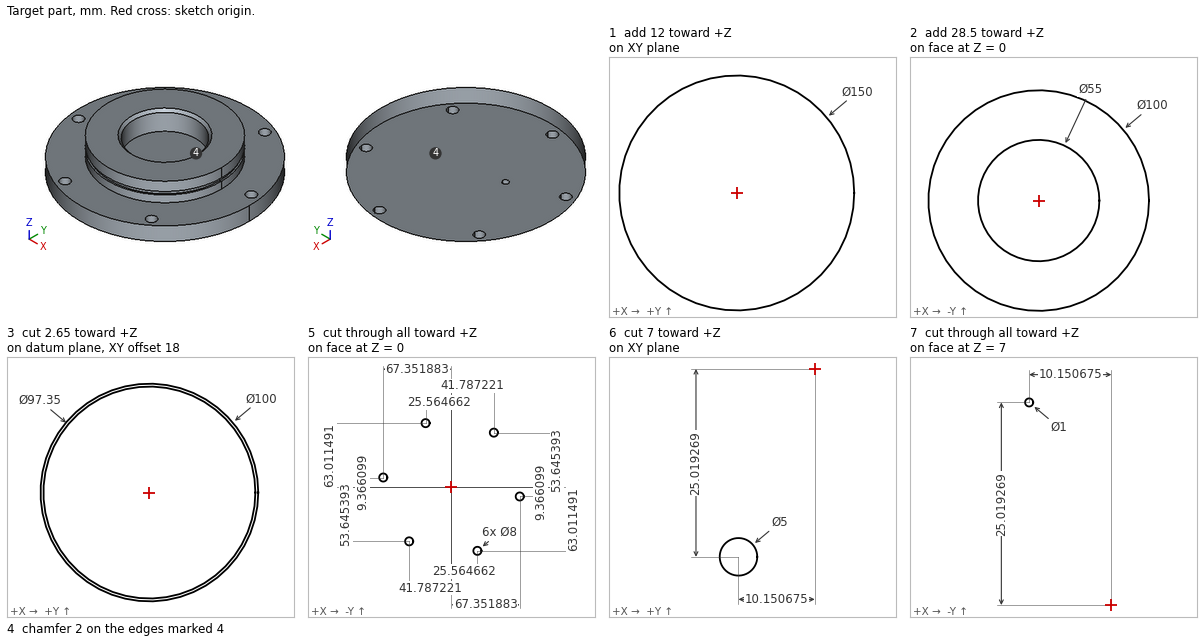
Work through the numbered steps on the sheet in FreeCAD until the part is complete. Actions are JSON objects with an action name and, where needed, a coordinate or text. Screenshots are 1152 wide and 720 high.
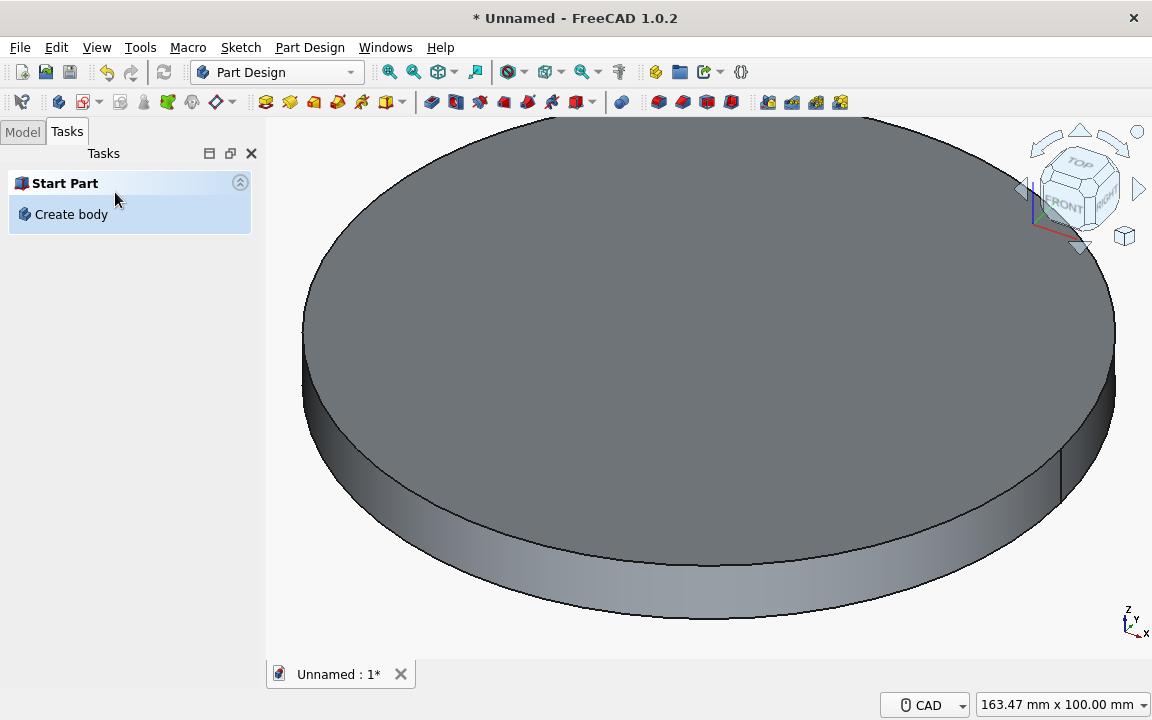
{"action": "left_click", "coordinate": [390, 72]}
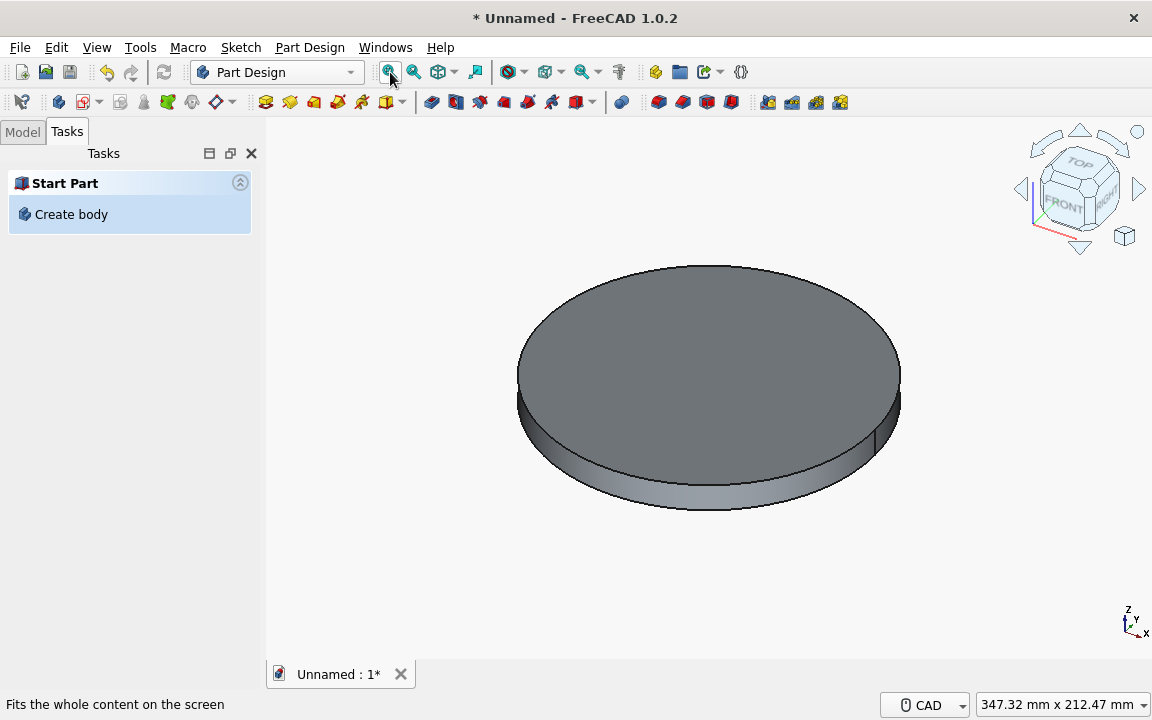
{"action": "key", "text": "5"}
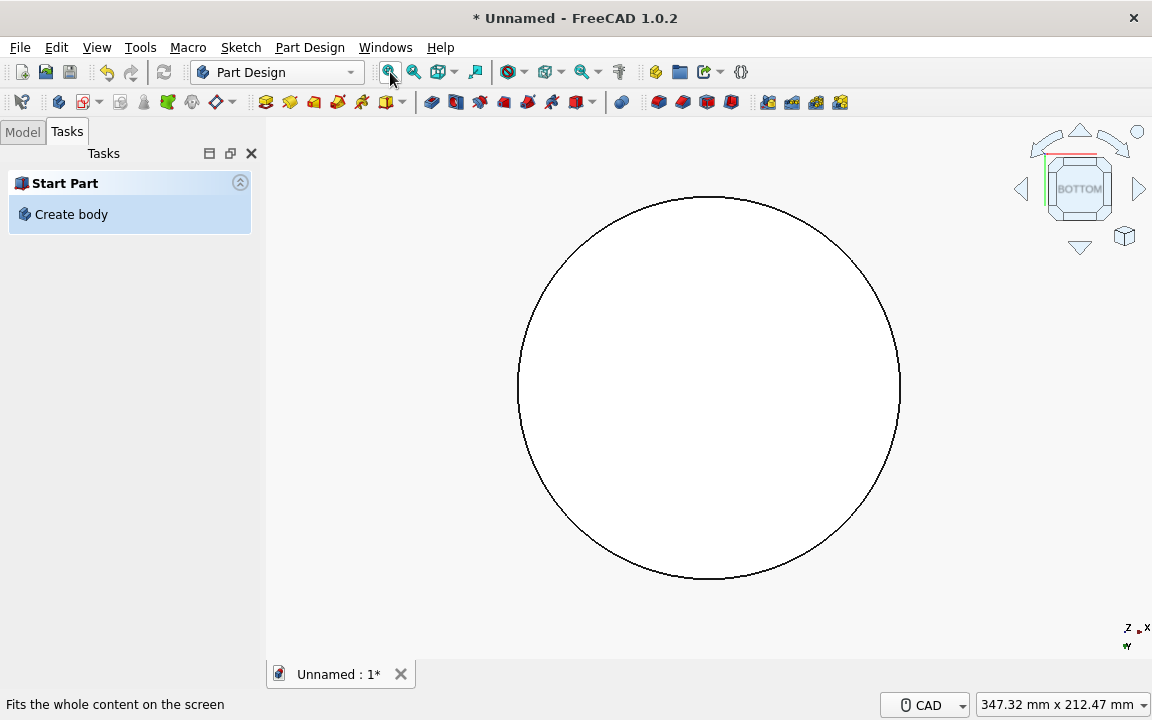
{"action": "left_click", "coordinate": [709, 387]}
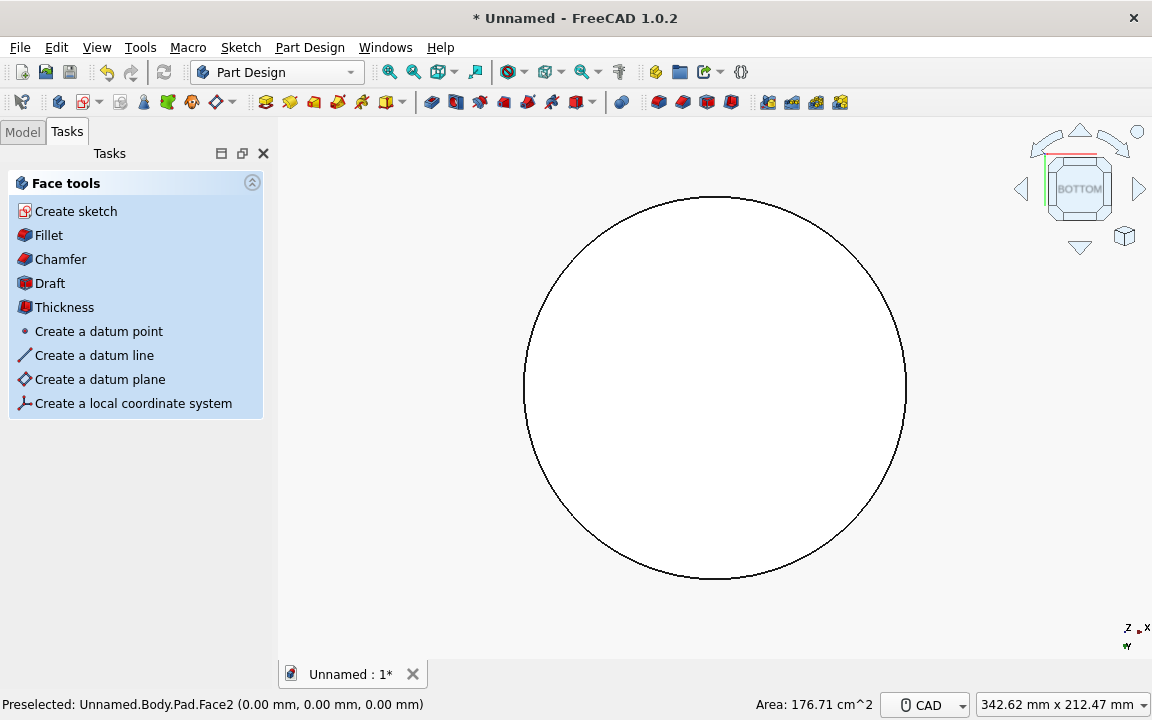
{"action": "left_click", "coordinate": [84, 102]}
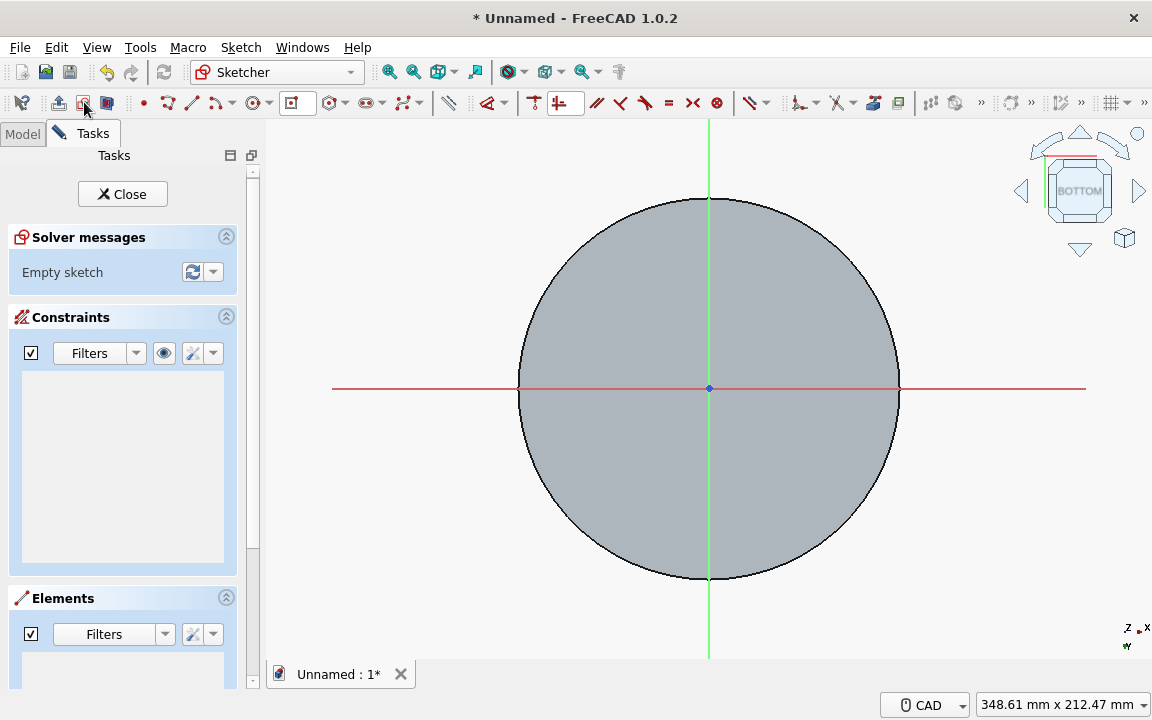
{"action": "left_click", "coordinate": [254, 104]}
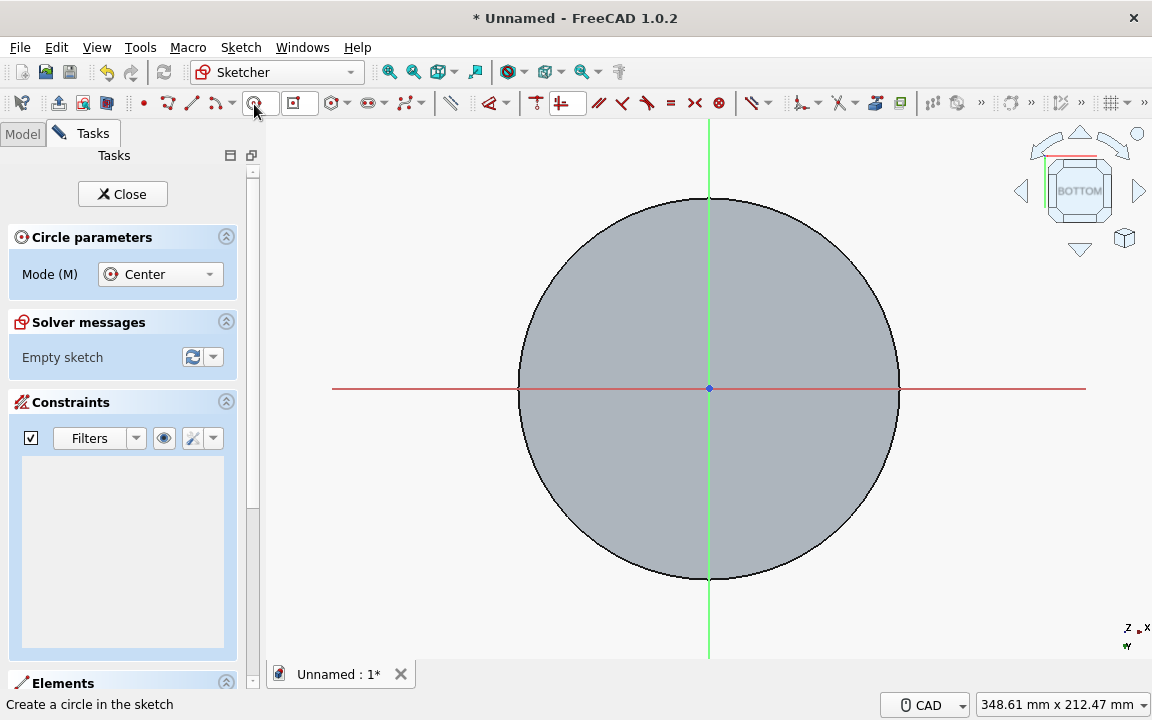
{"action": "left_click", "coordinate": [709, 389]}
{"action": "mouse_move", "coordinate": [799, 299]}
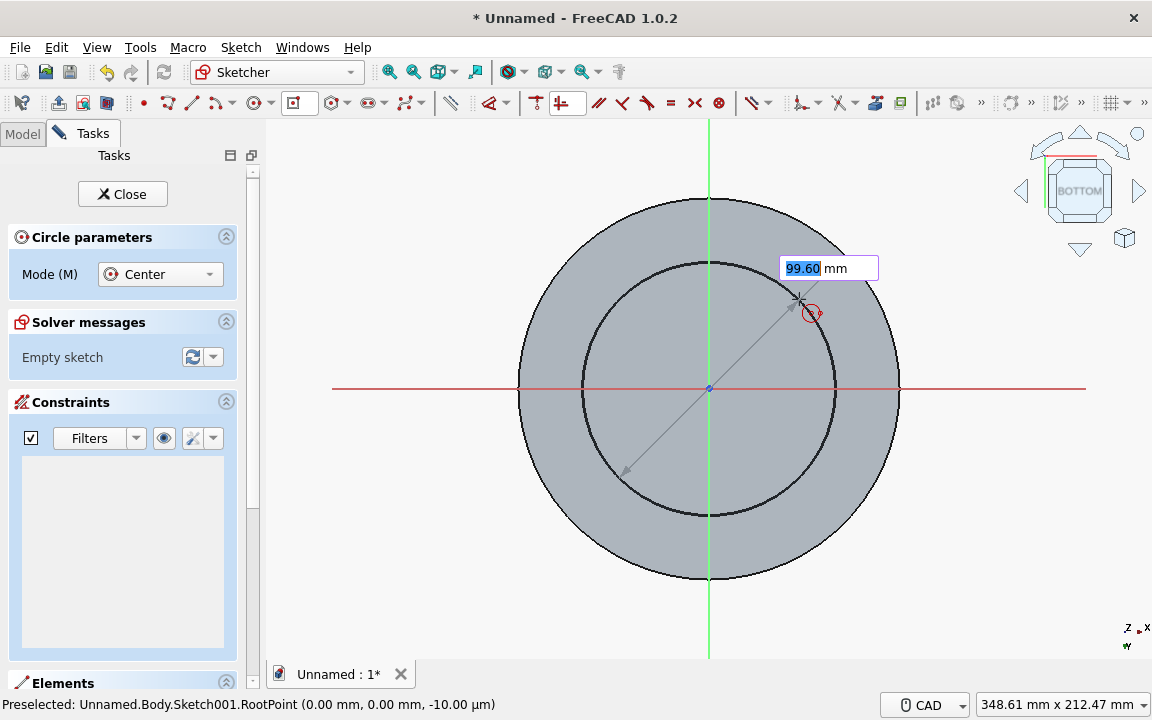
{"action": "type", "text": "100"}
{"action": "key", "text": "Return"}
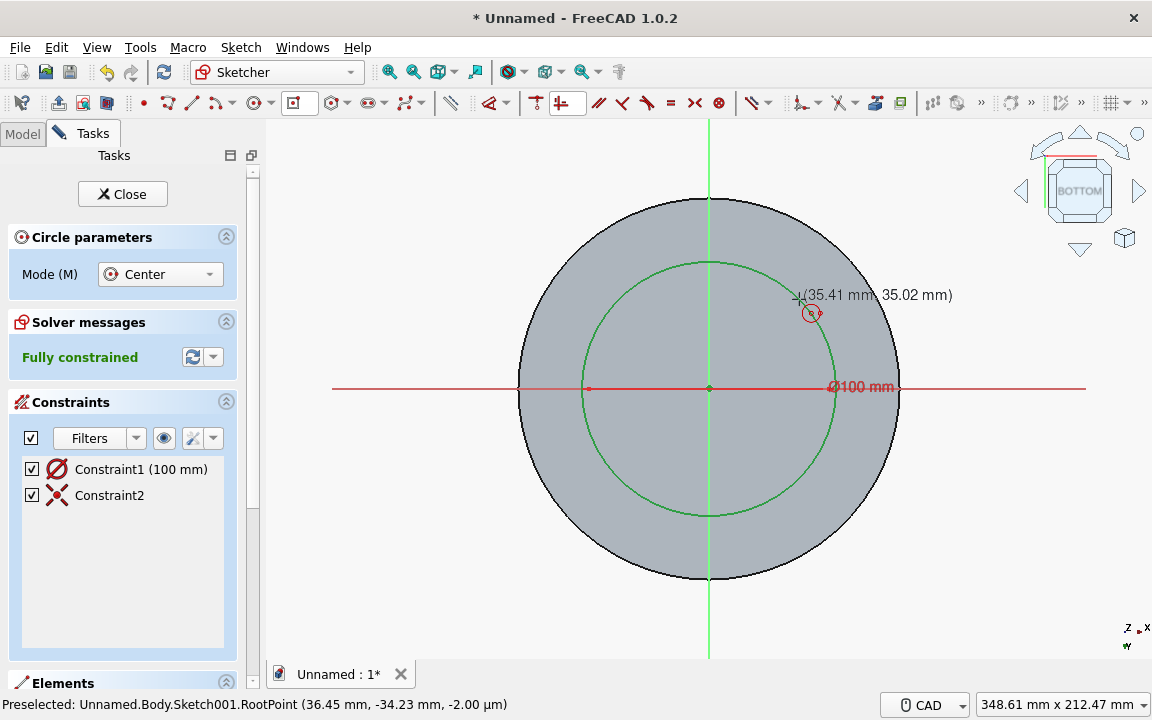
{"action": "left_click", "coordinate": [709, 389]}
{"action": "mouse_move", "coordinate": [758, 340]}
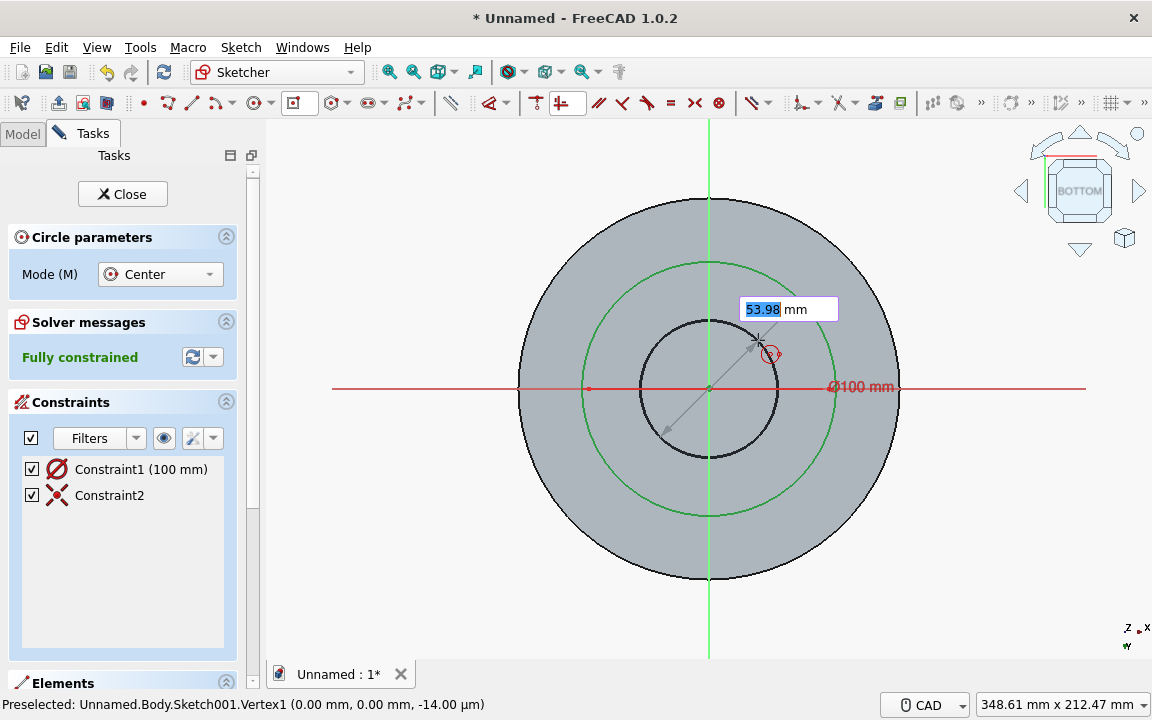
{"action": "type", "text": "55"}
{"action": "key", "text": "Return"}
{"action": "key", "text": "Escape"}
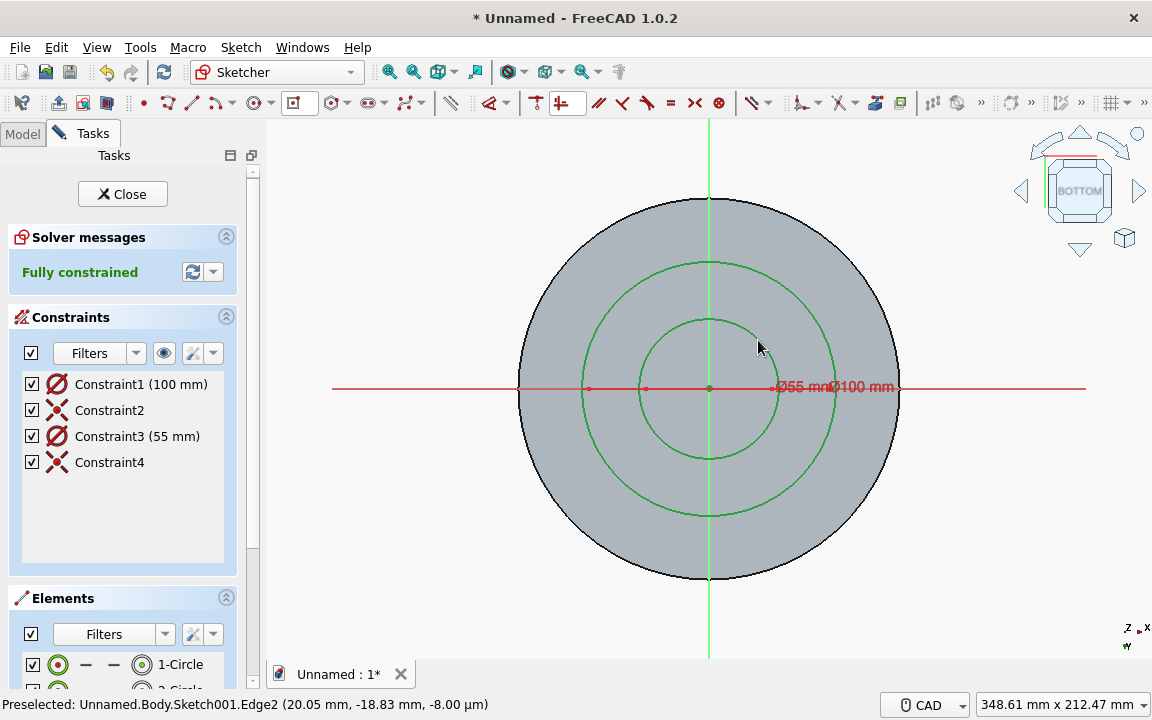
{"action": "left_click", "coordinate": [123, 194]}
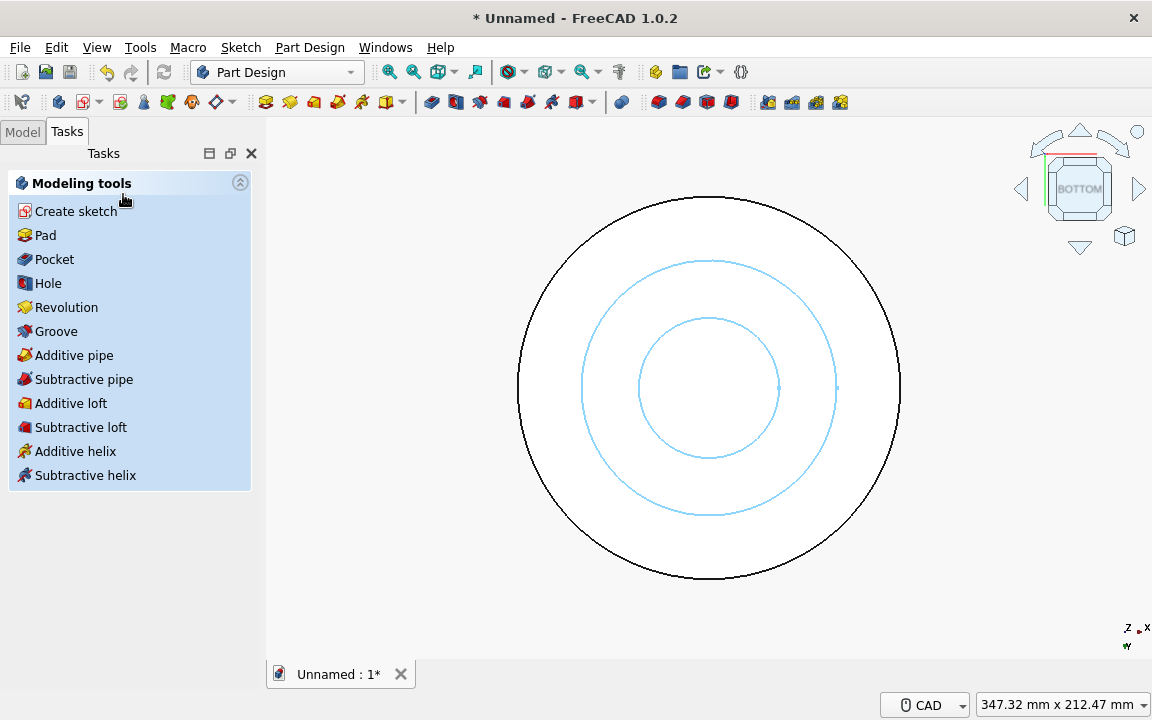
{"action": "left_click", "coordinate": [266, 102]}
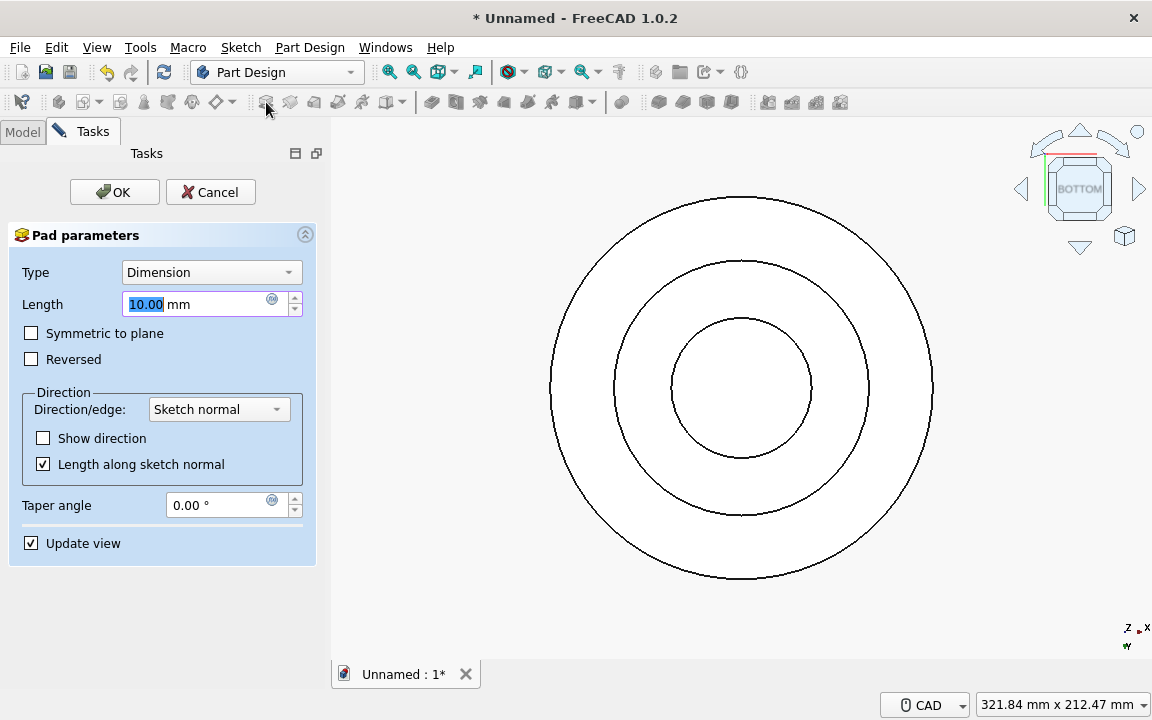
{"action": "type", "text": "28.5"}
{"action": "key", "text": "Tab"}